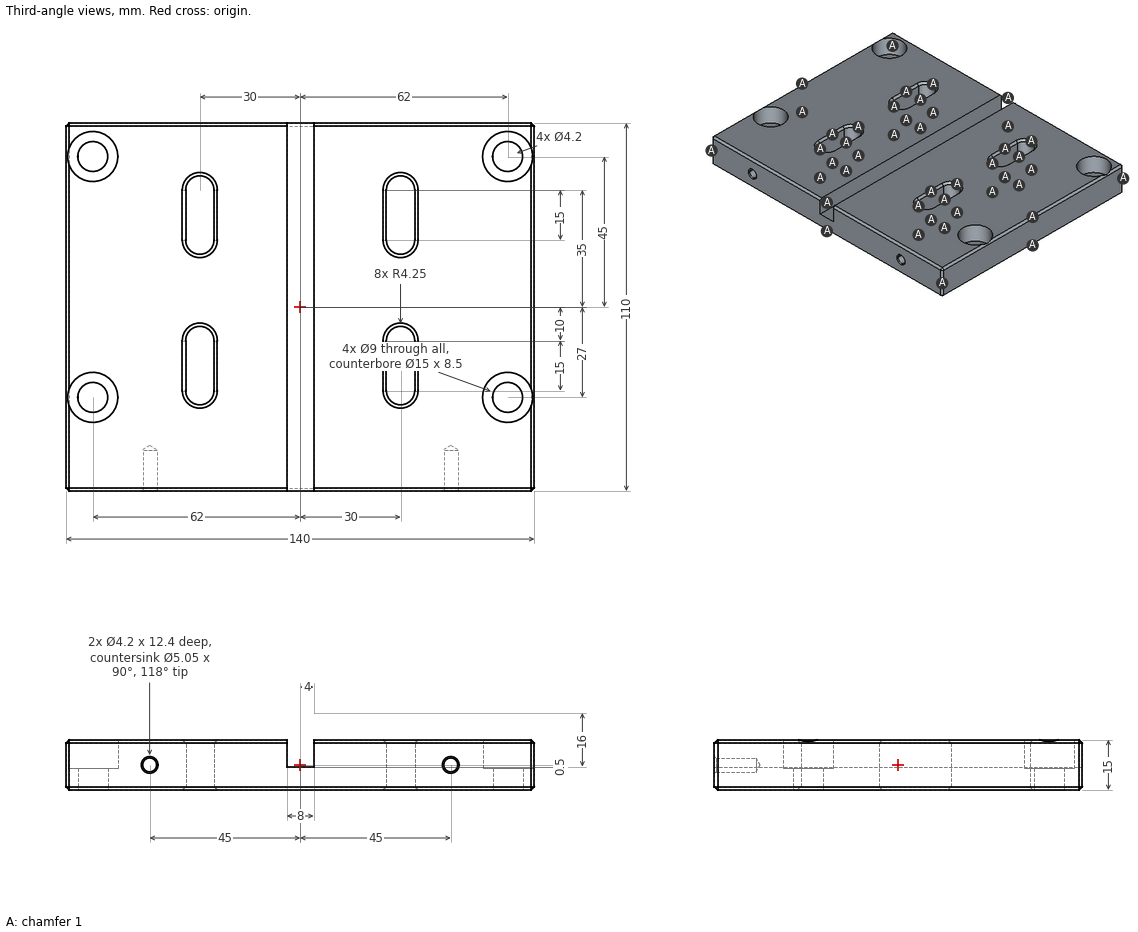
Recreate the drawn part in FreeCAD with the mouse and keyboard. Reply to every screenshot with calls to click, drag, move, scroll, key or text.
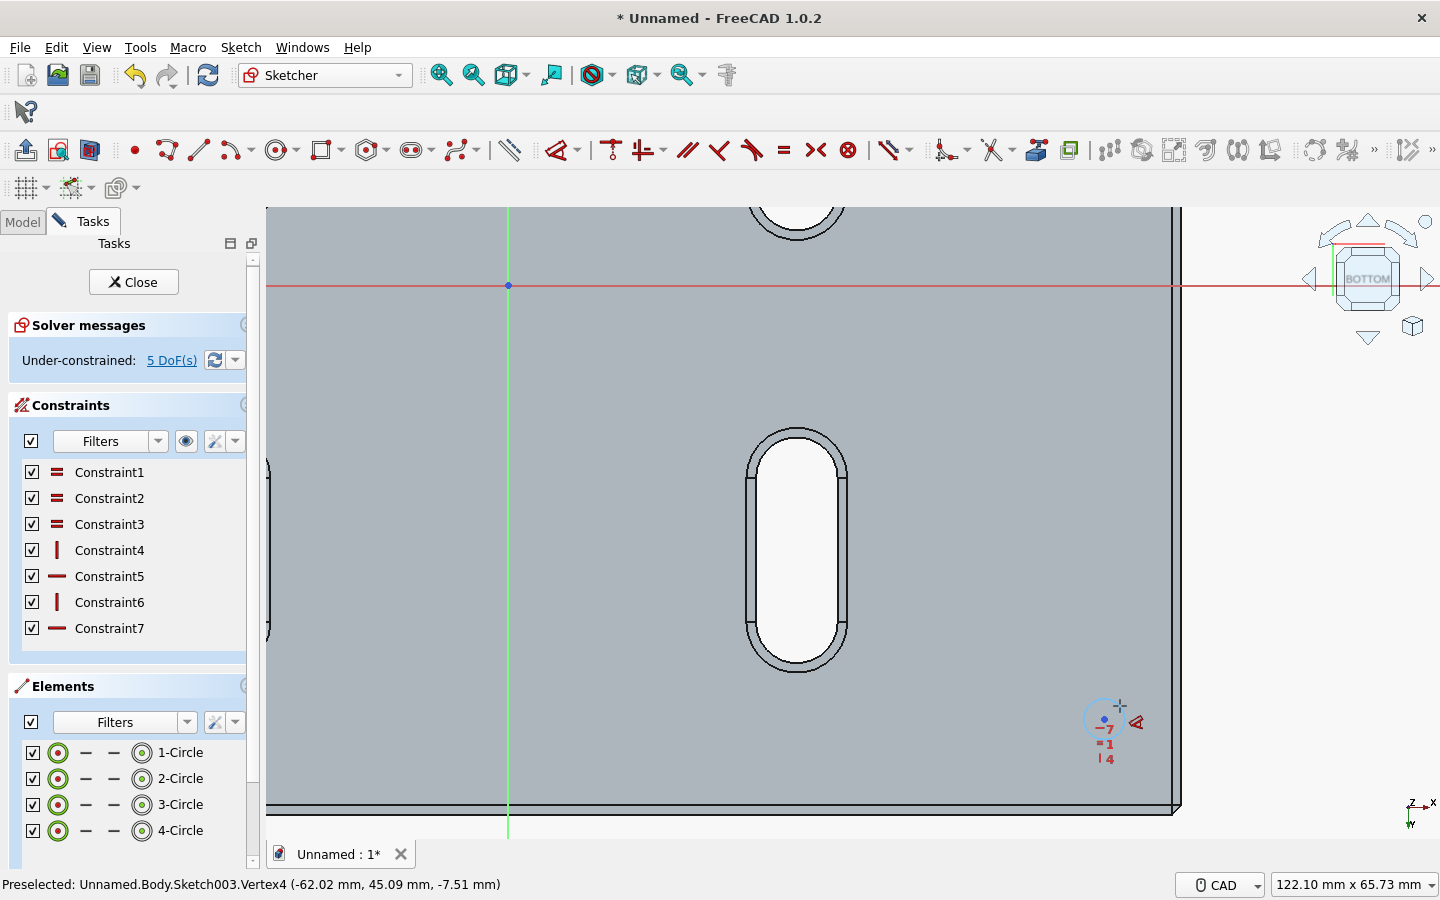
click(1119, 705)
click(1142, 683)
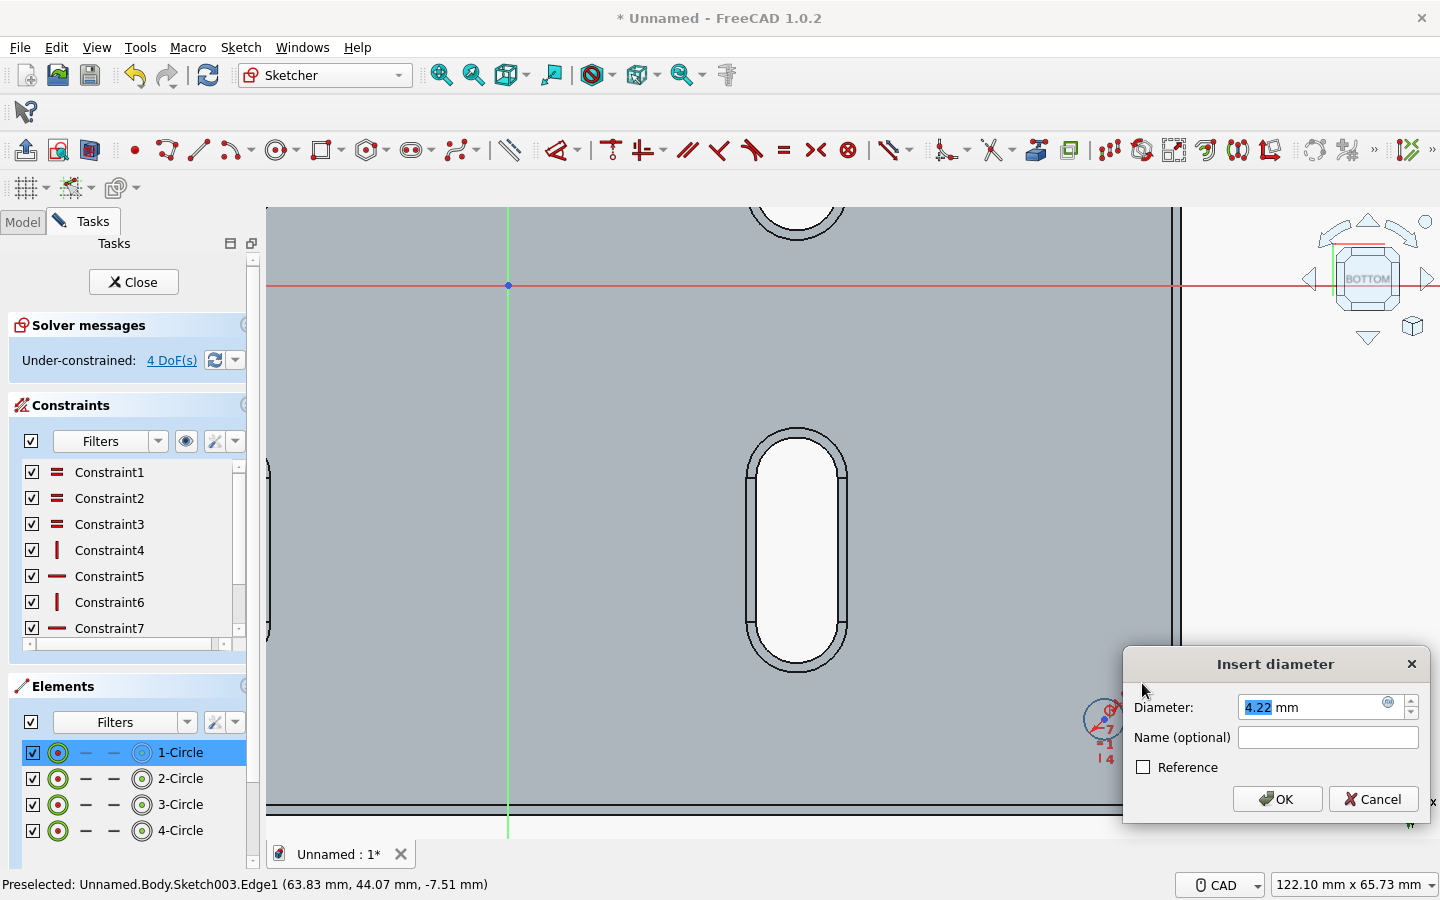
text(4.2)
key(Return)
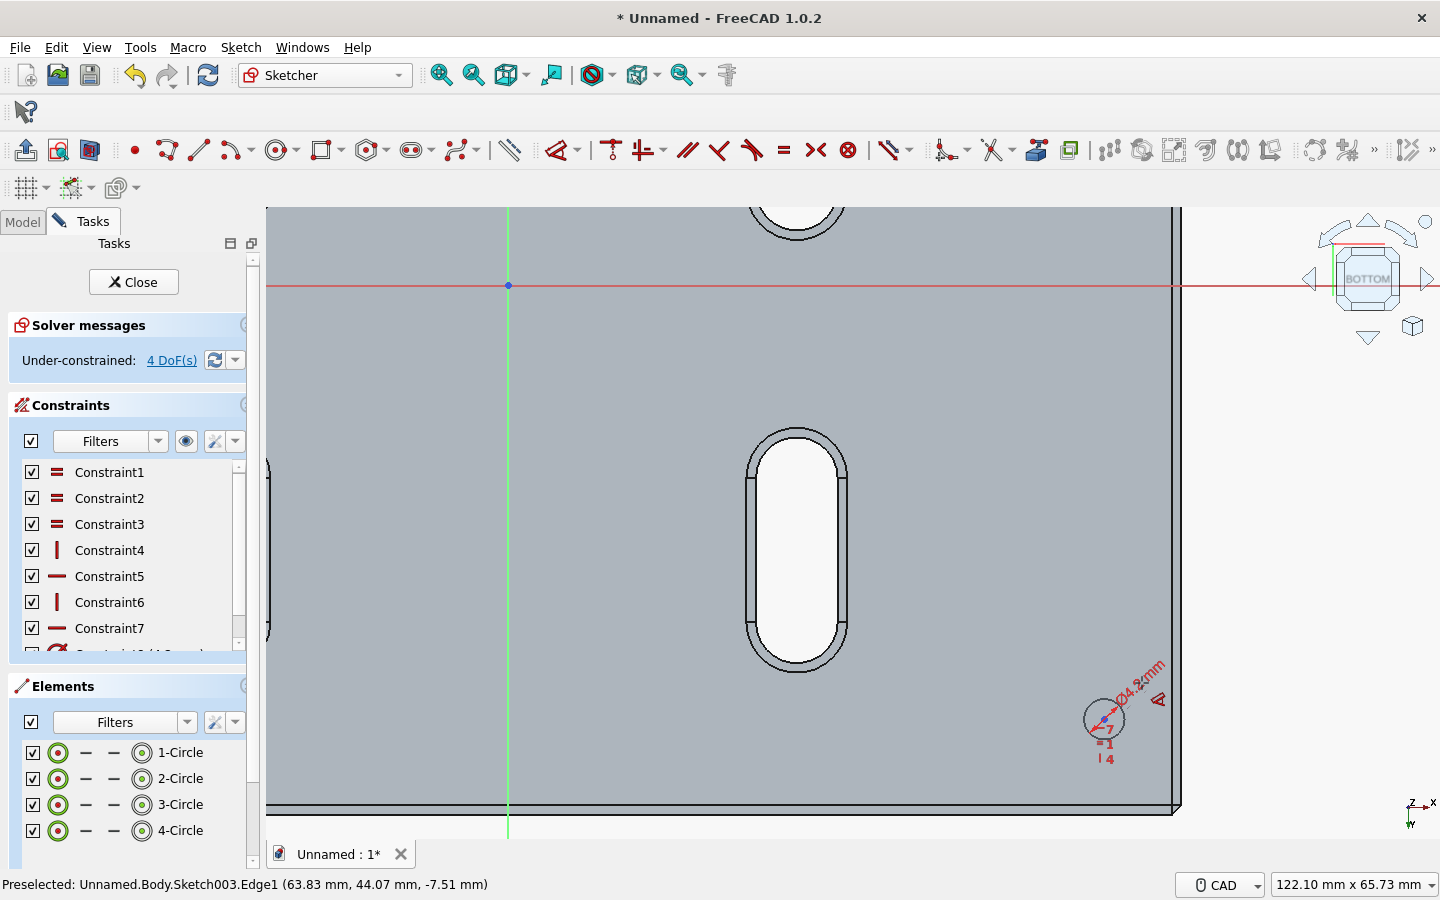
click(1104, 719)
click(806, 753)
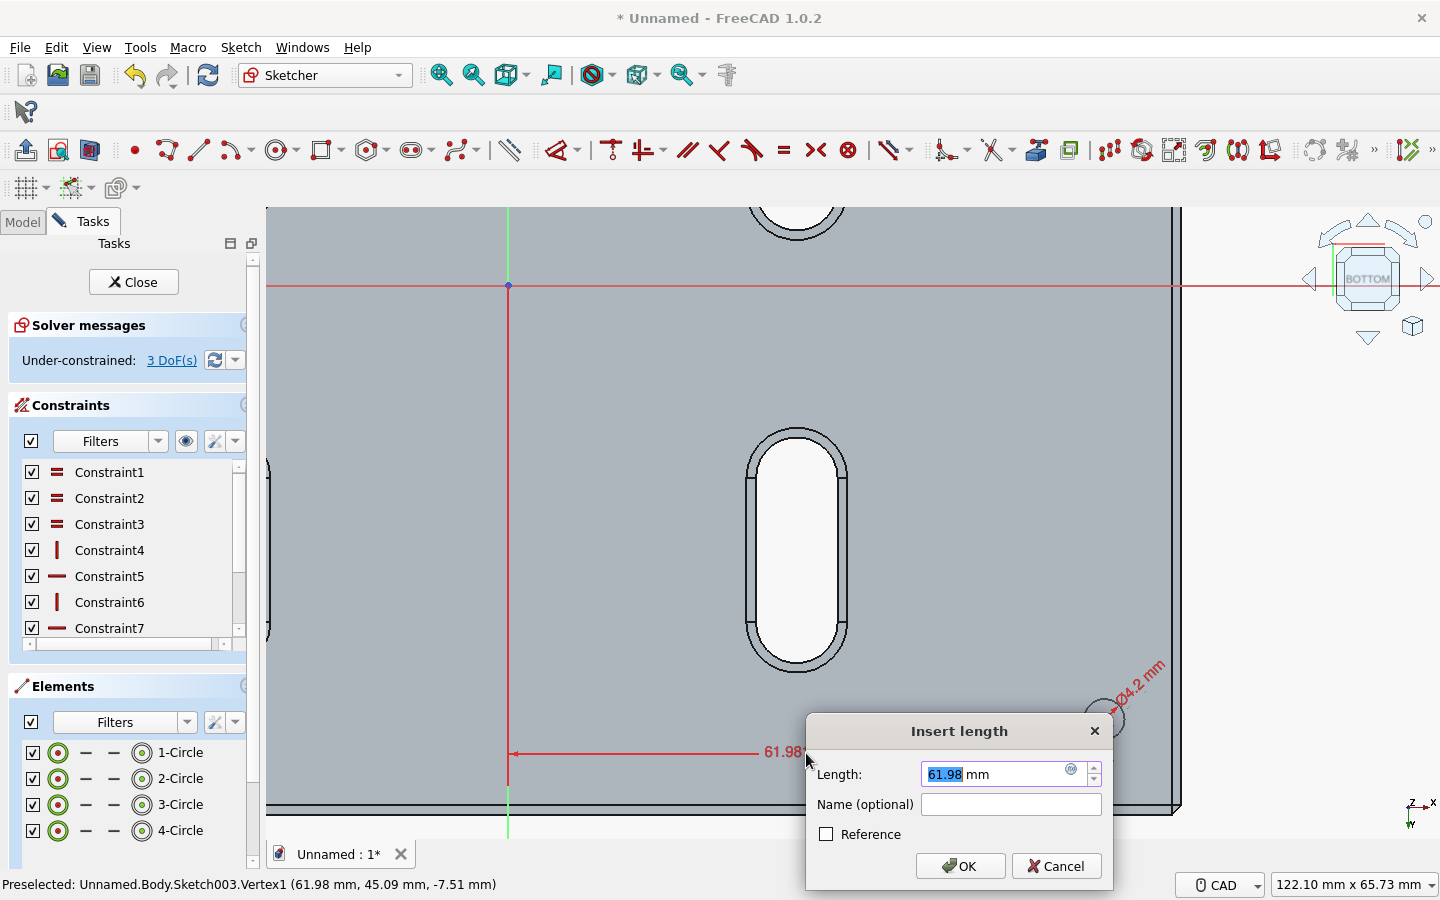
text(62)
key(Return)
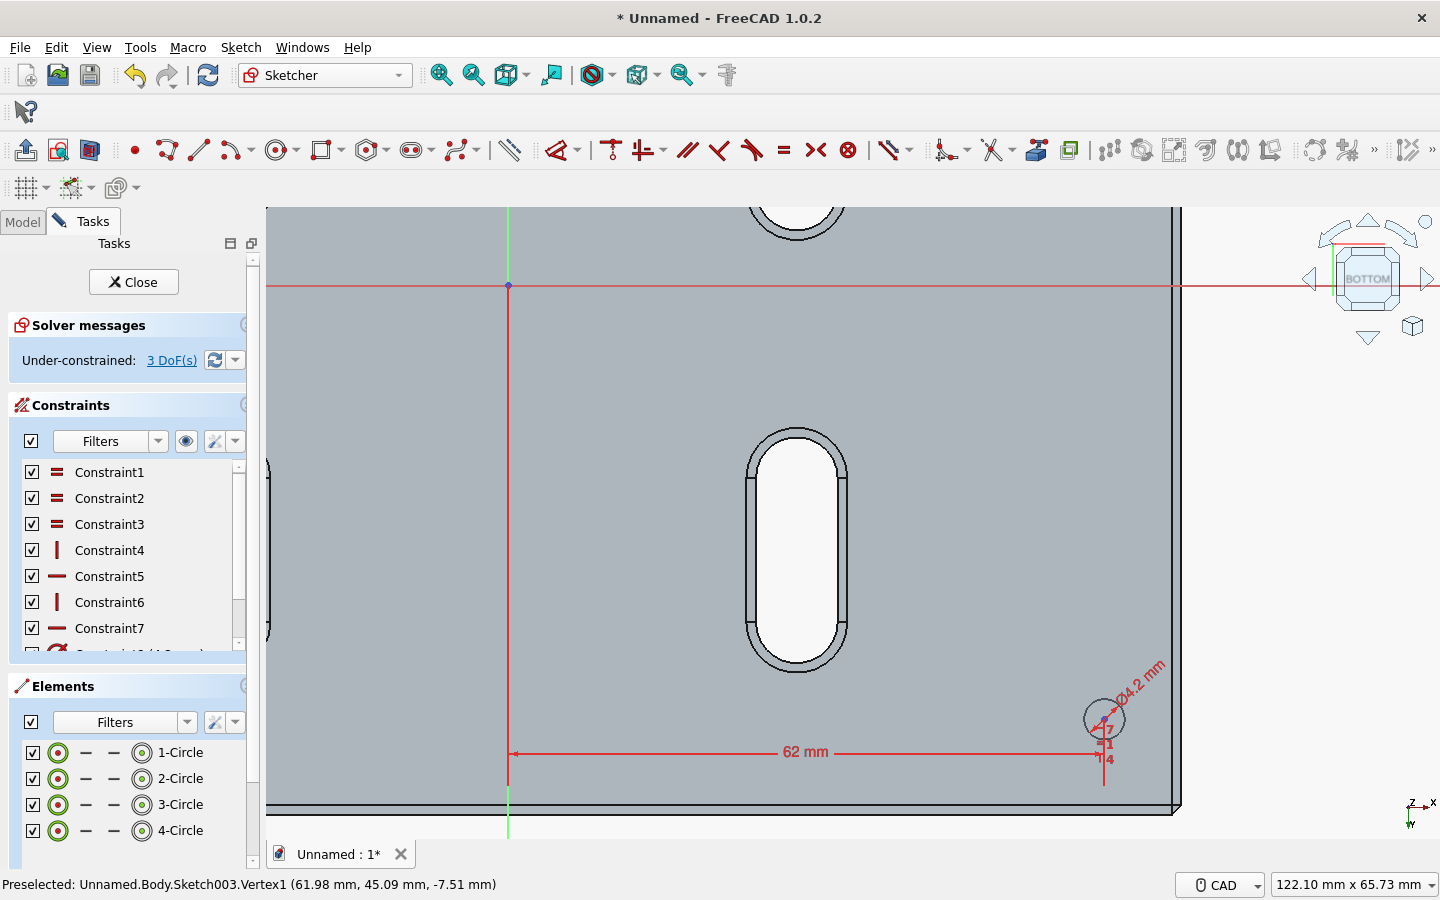
click(1105, 719)
click(1139, 503)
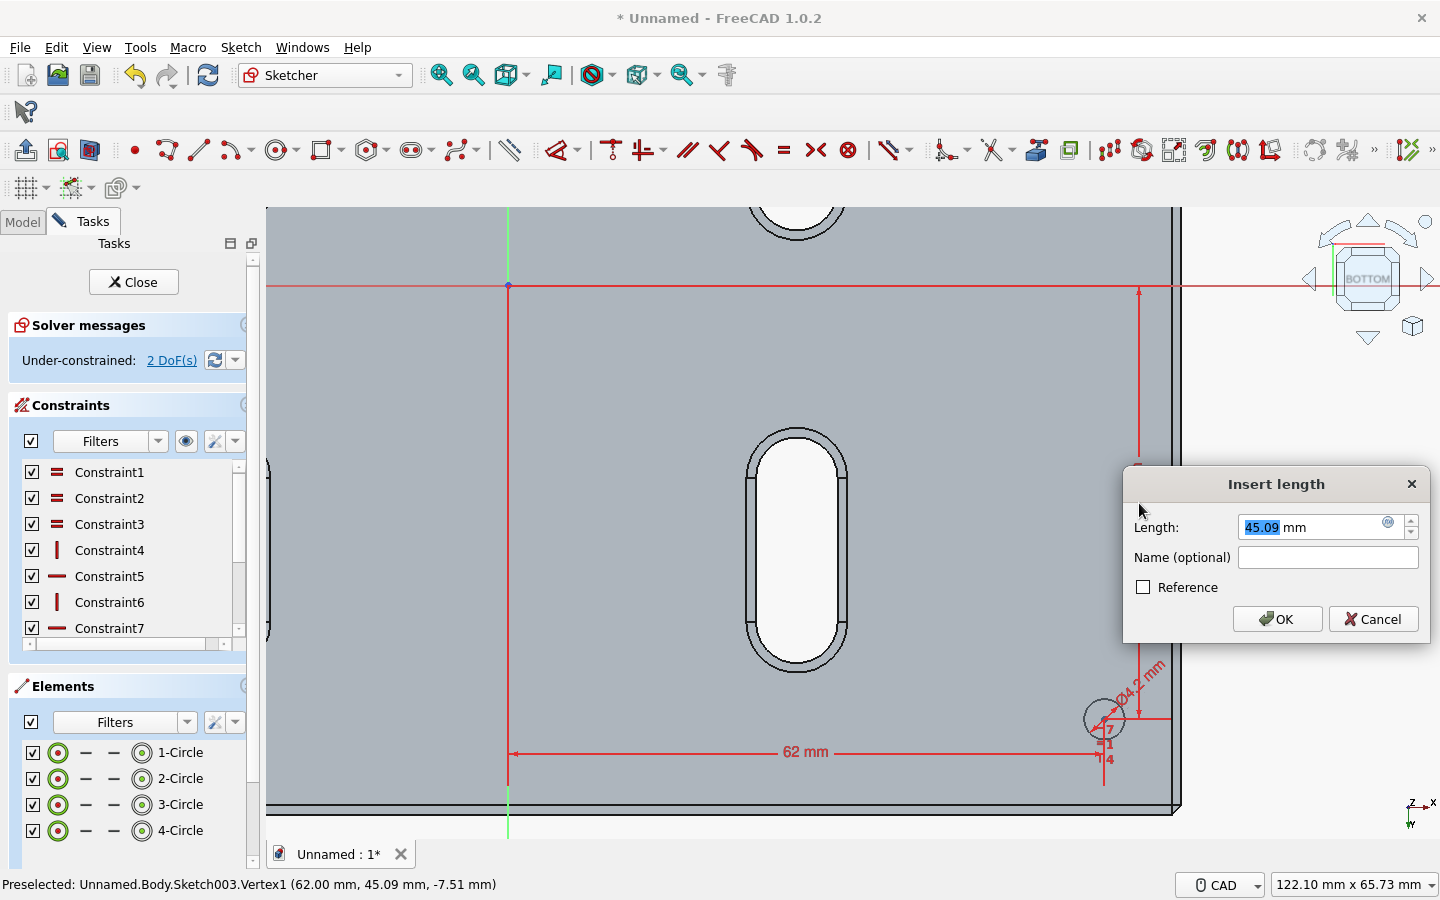
text(45)
key(Return)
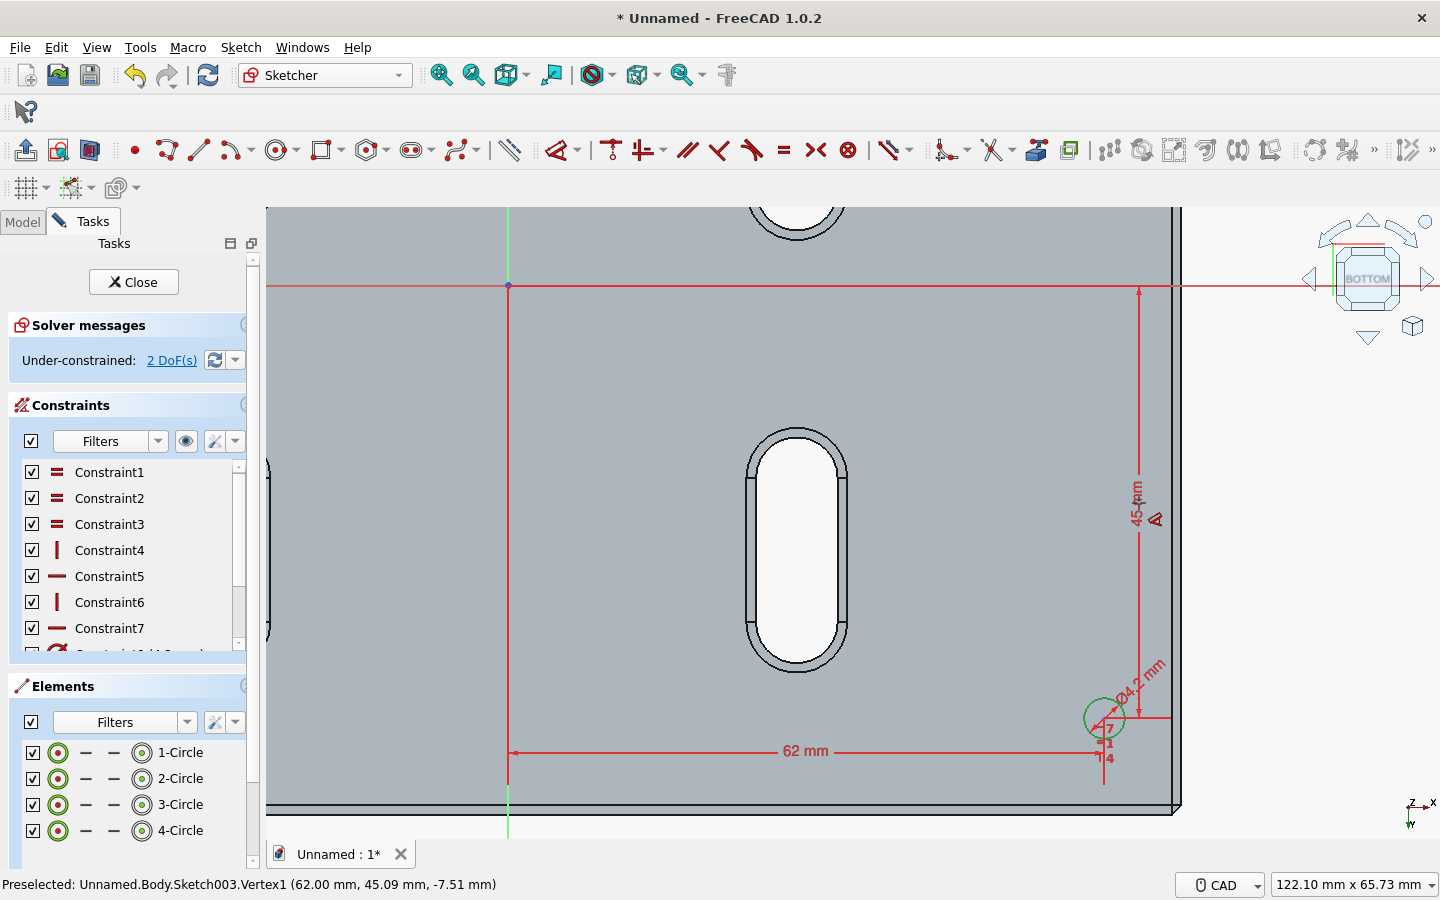
scroll(1120, 706, down, 3)